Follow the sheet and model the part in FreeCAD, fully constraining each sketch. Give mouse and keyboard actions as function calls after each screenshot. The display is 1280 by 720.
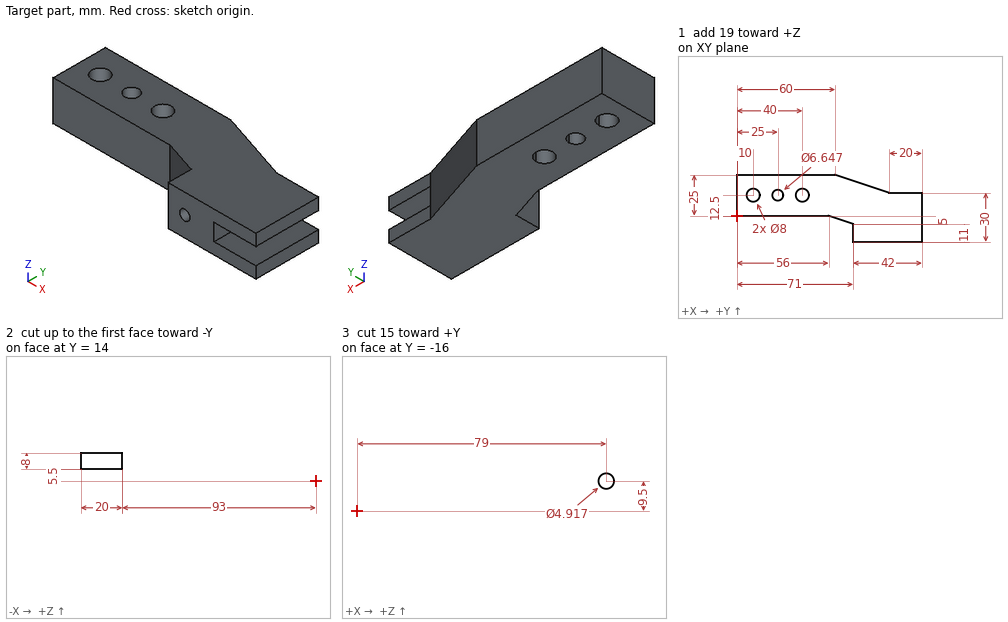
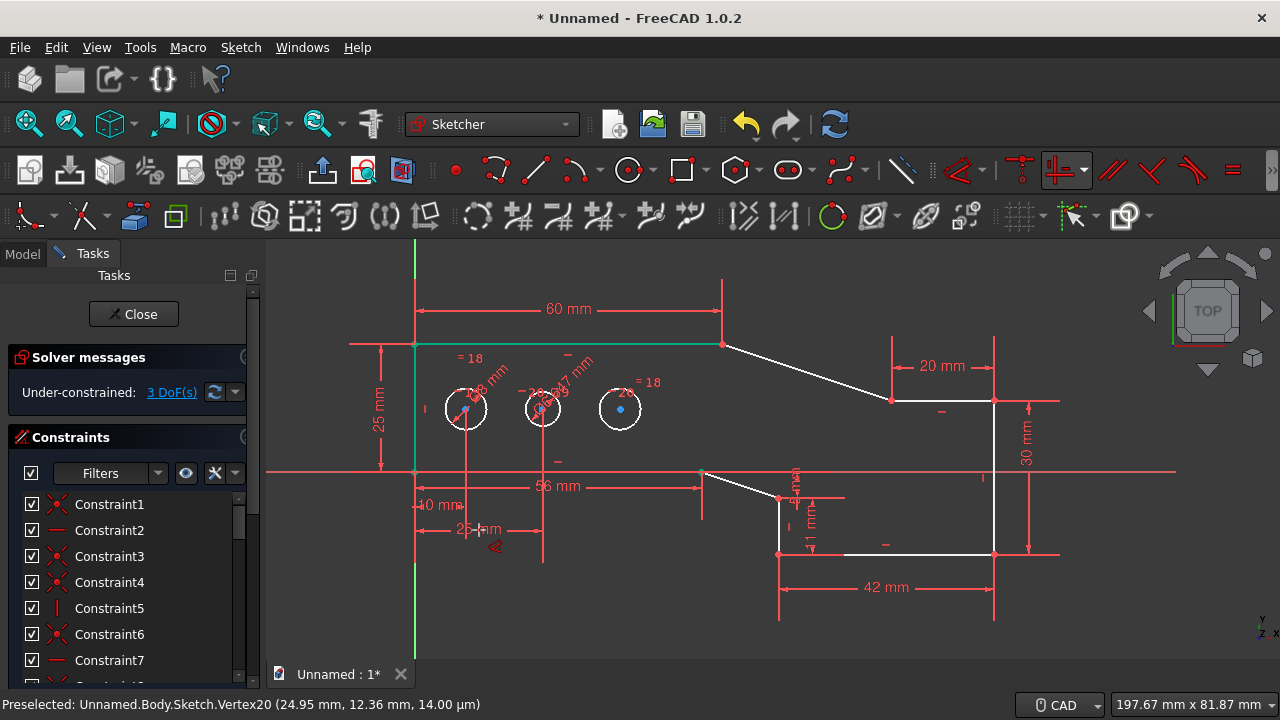
click(620, 409)
click(565, 530)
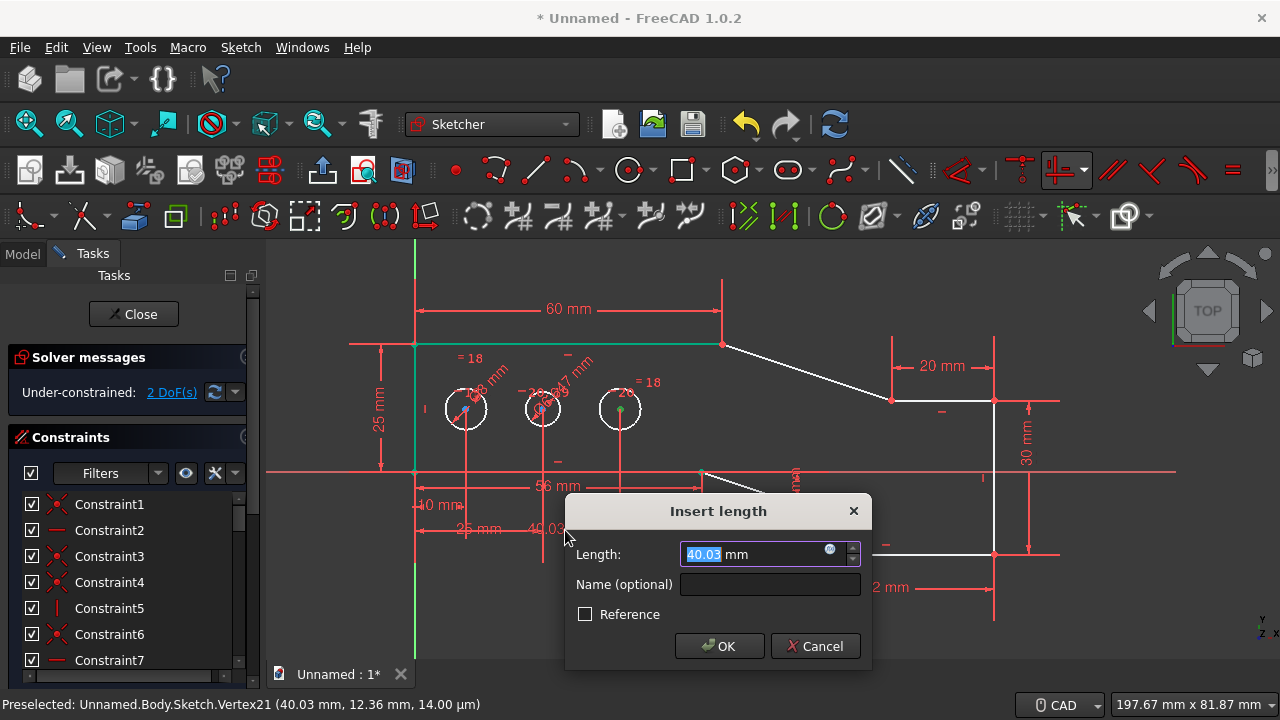
text(40)
key(Return)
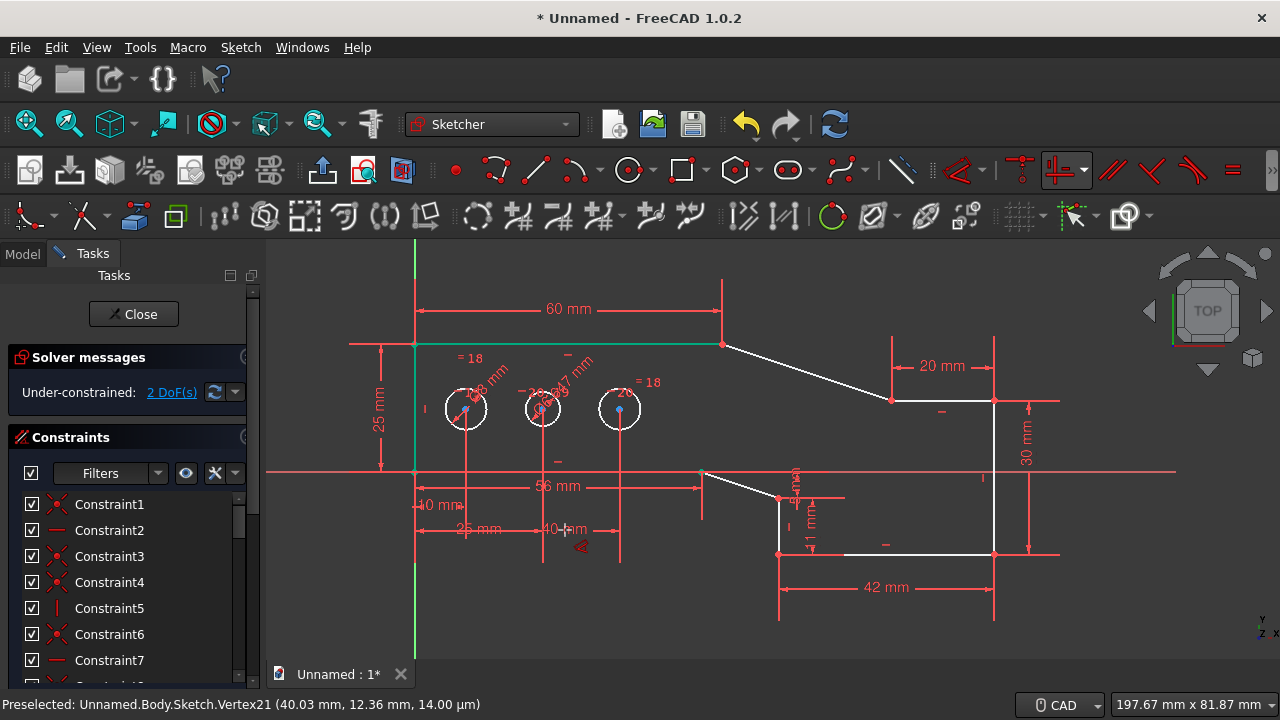
click(779, 498)
click(680, 532)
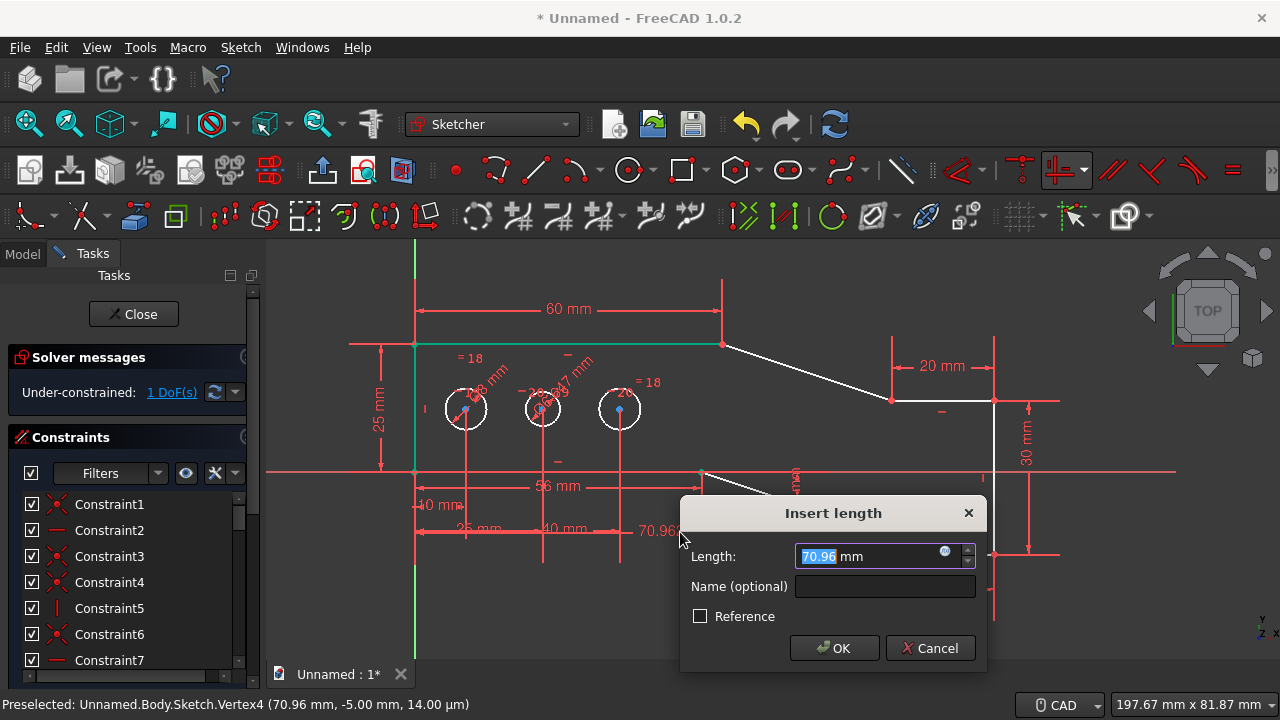
text(71)
key(Return)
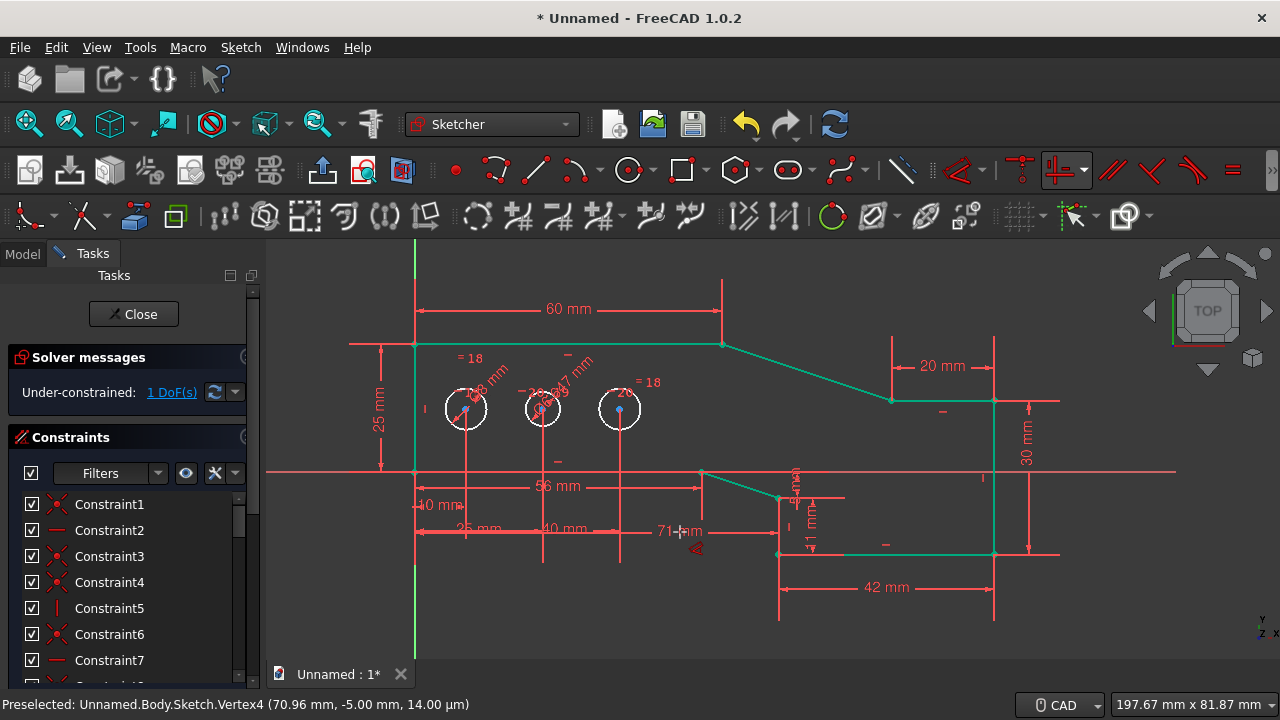
click(466, 409)
click(381, 441)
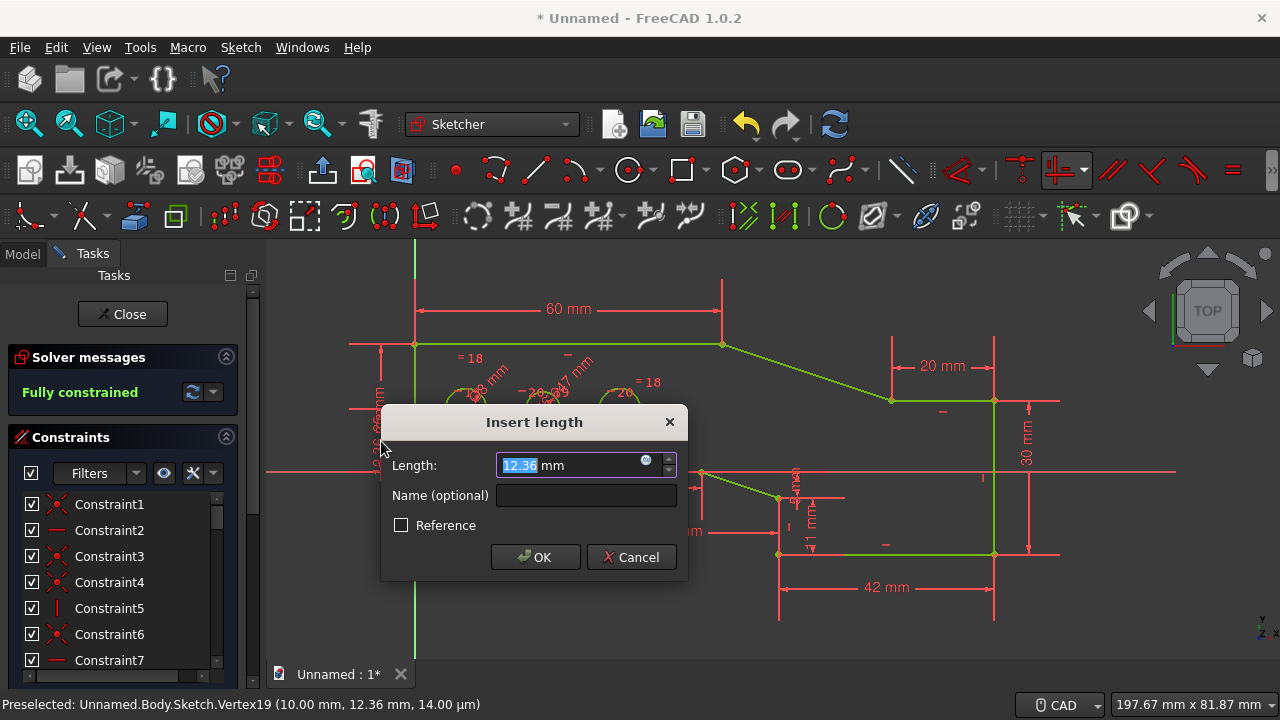
text(12.5)
key(Return)
key(Escape)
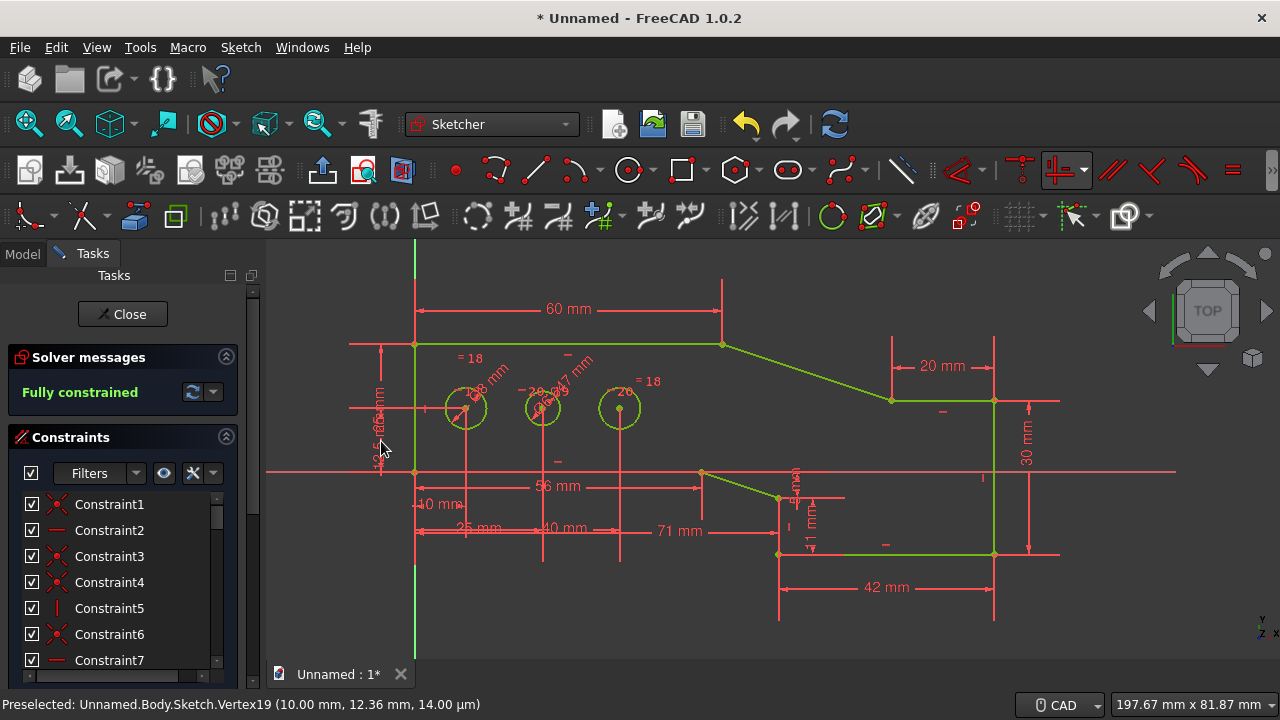
click(123, 314)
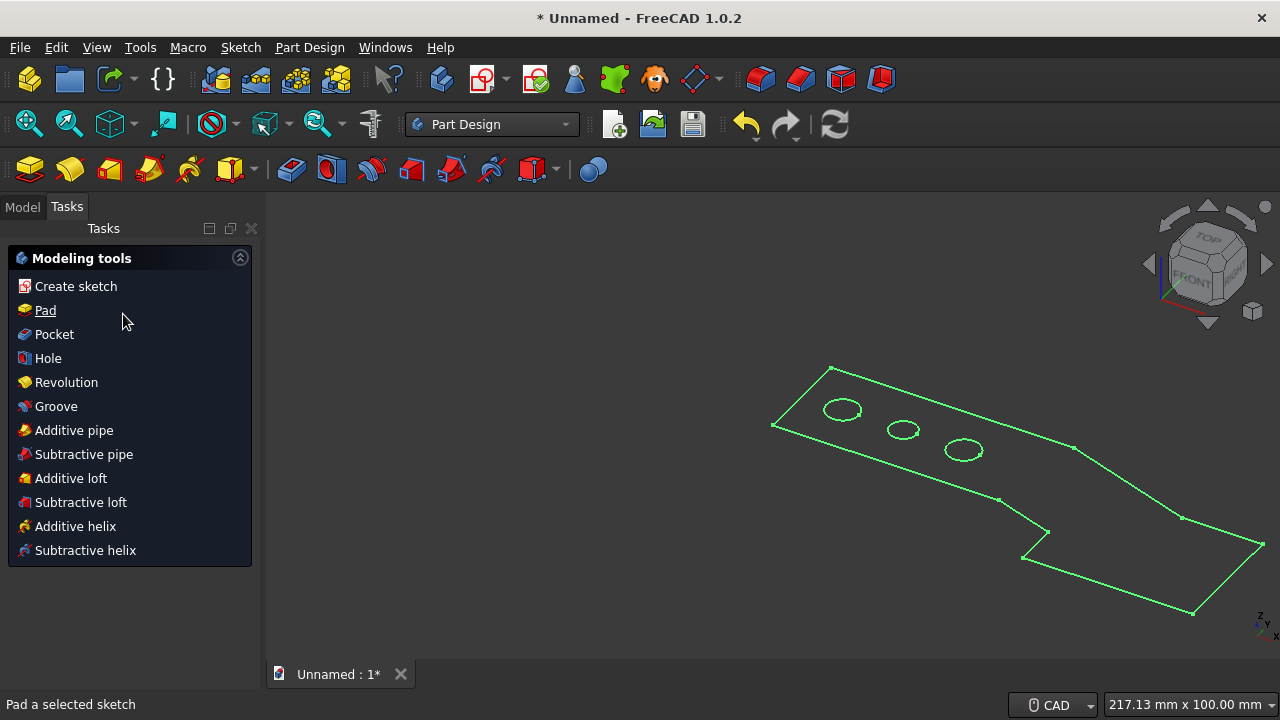
click(30, 170)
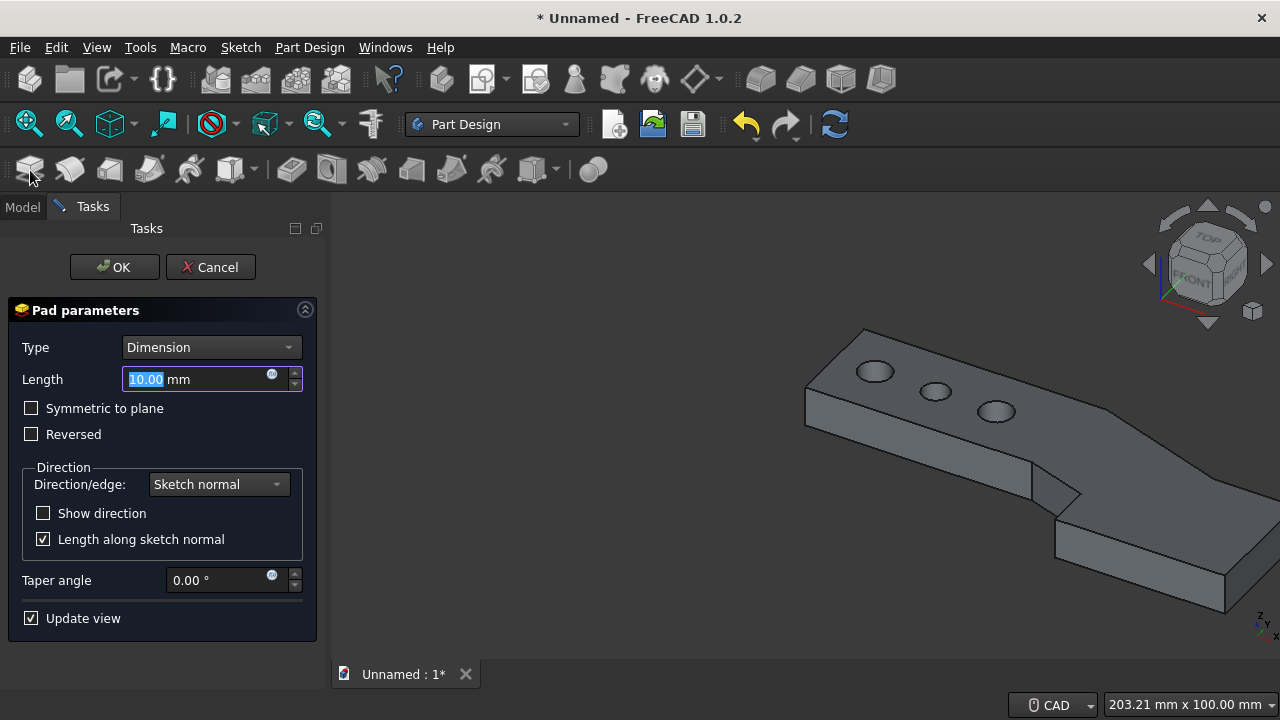
text(19)
key(Tab)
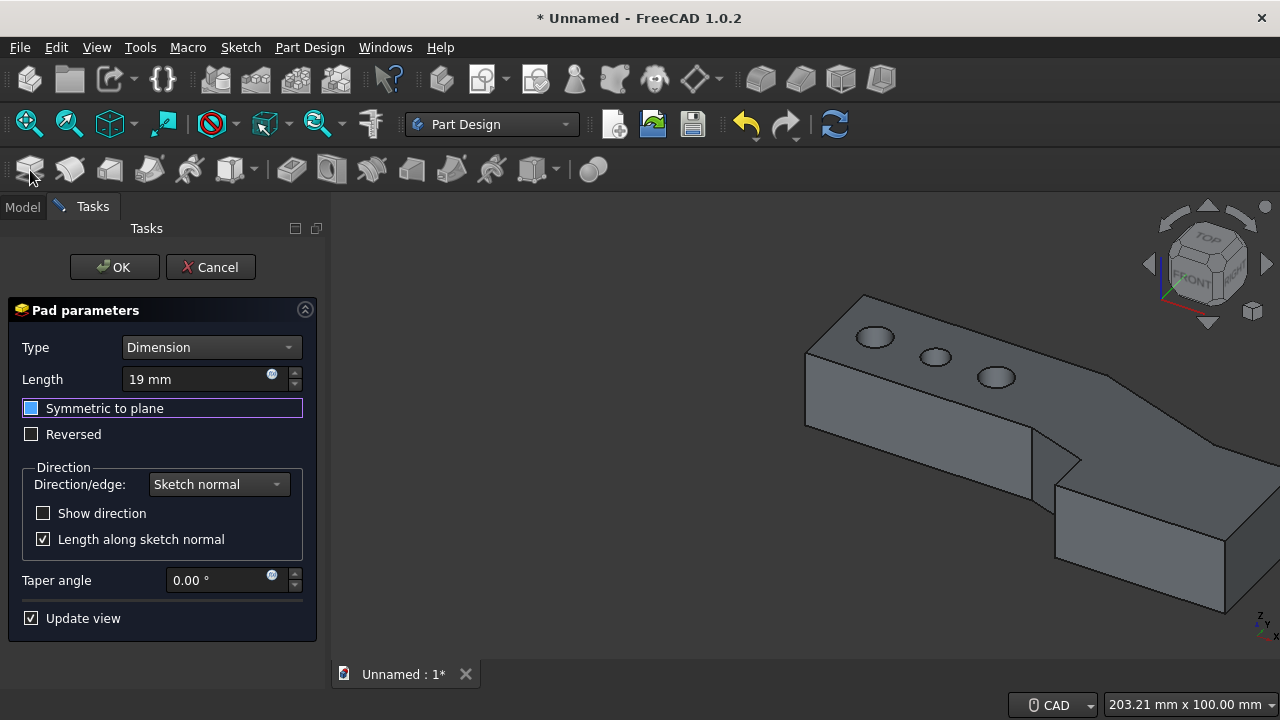
click(115, 267)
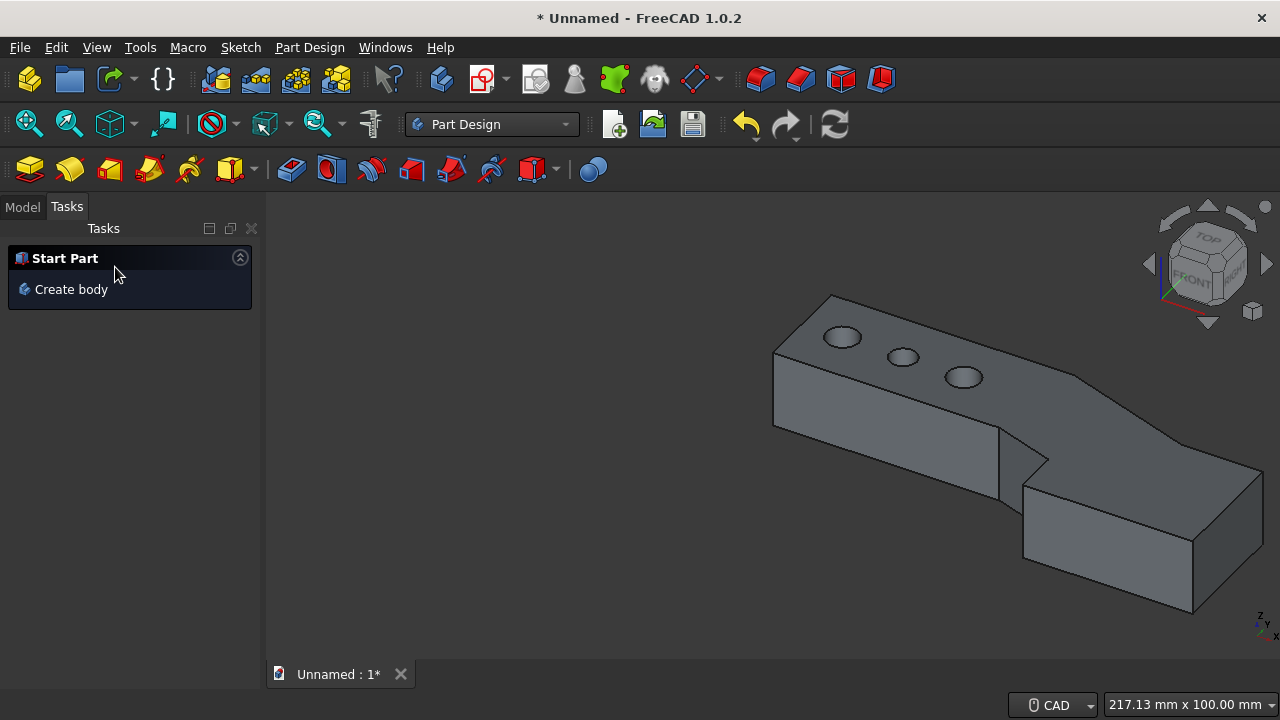
key(v)
key(f)